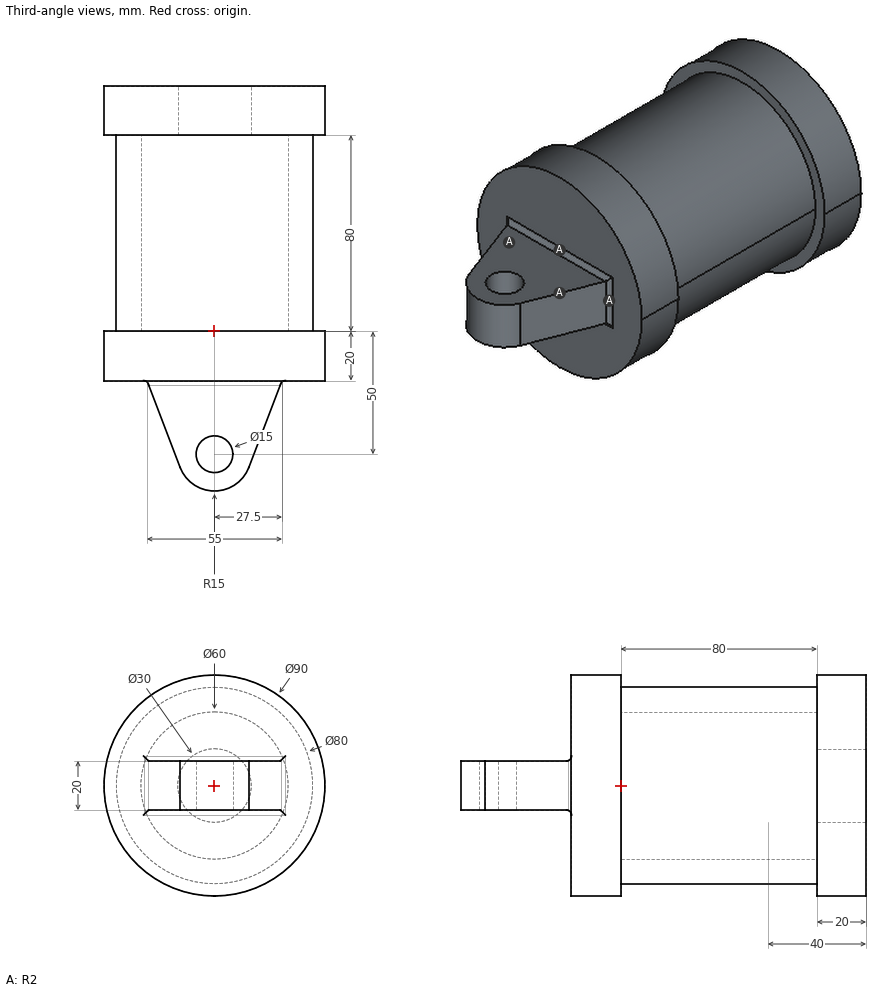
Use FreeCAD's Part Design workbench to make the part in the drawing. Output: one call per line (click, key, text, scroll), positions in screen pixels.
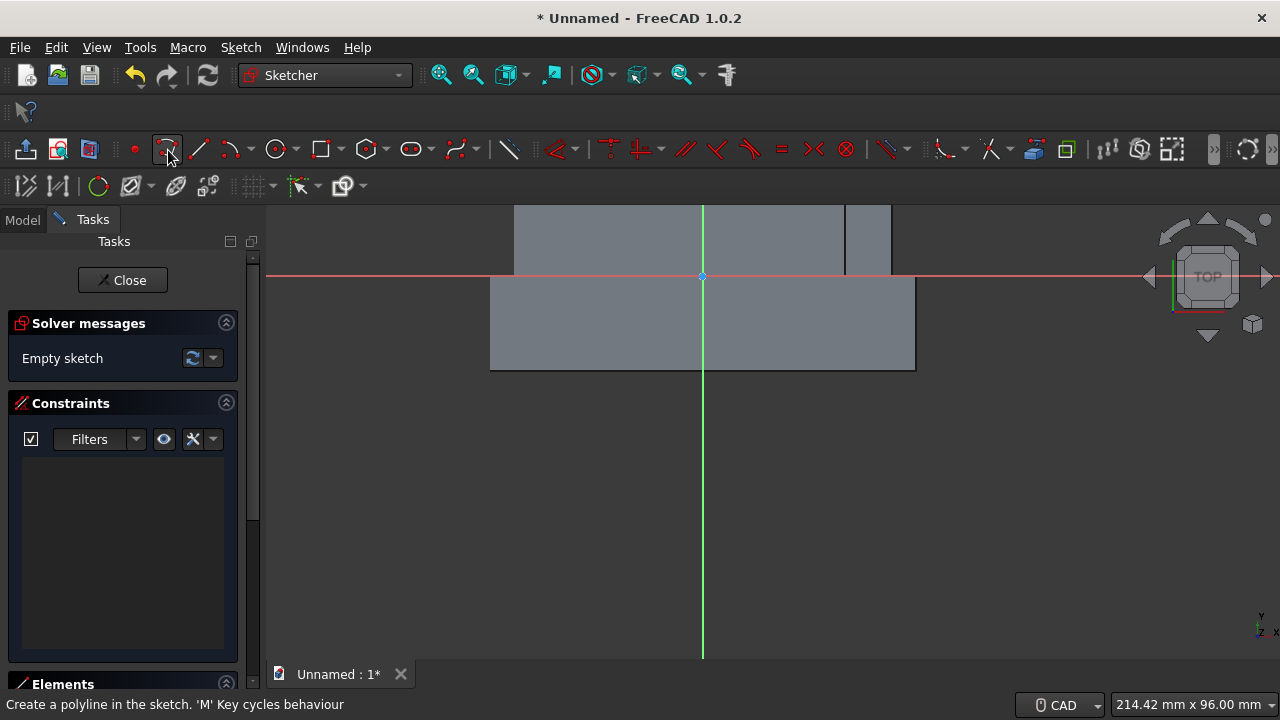
click(769, 538)
click(833, 371)
click(573, 371)
click(636, 538)
right_click(636, 538)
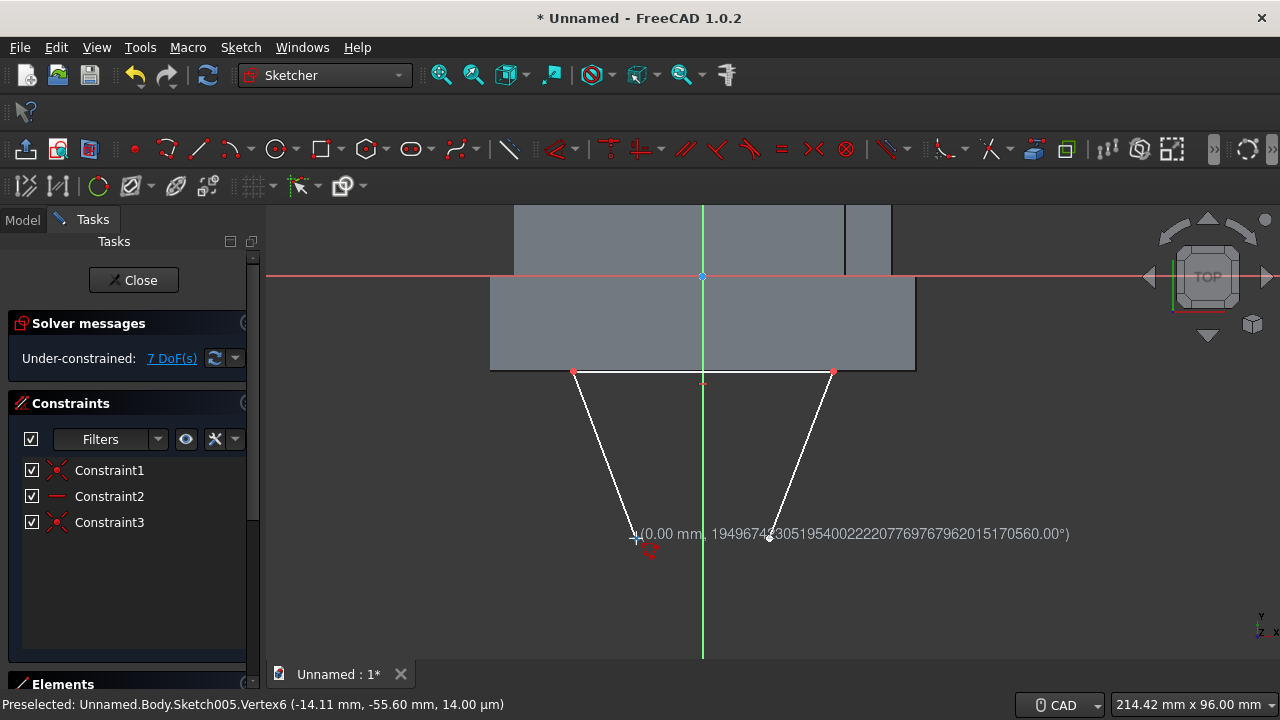
key(g)
key(3)
key(a)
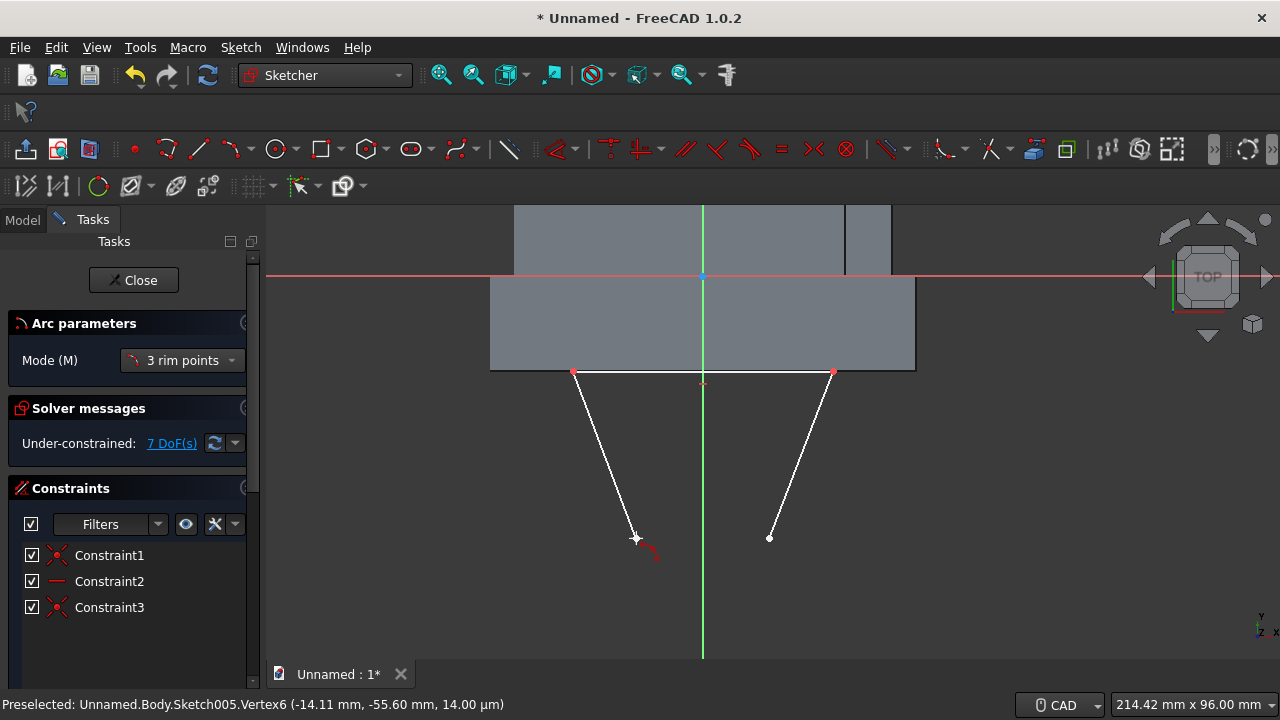
click(636, 539)
click(769, 539)
click(686, 581)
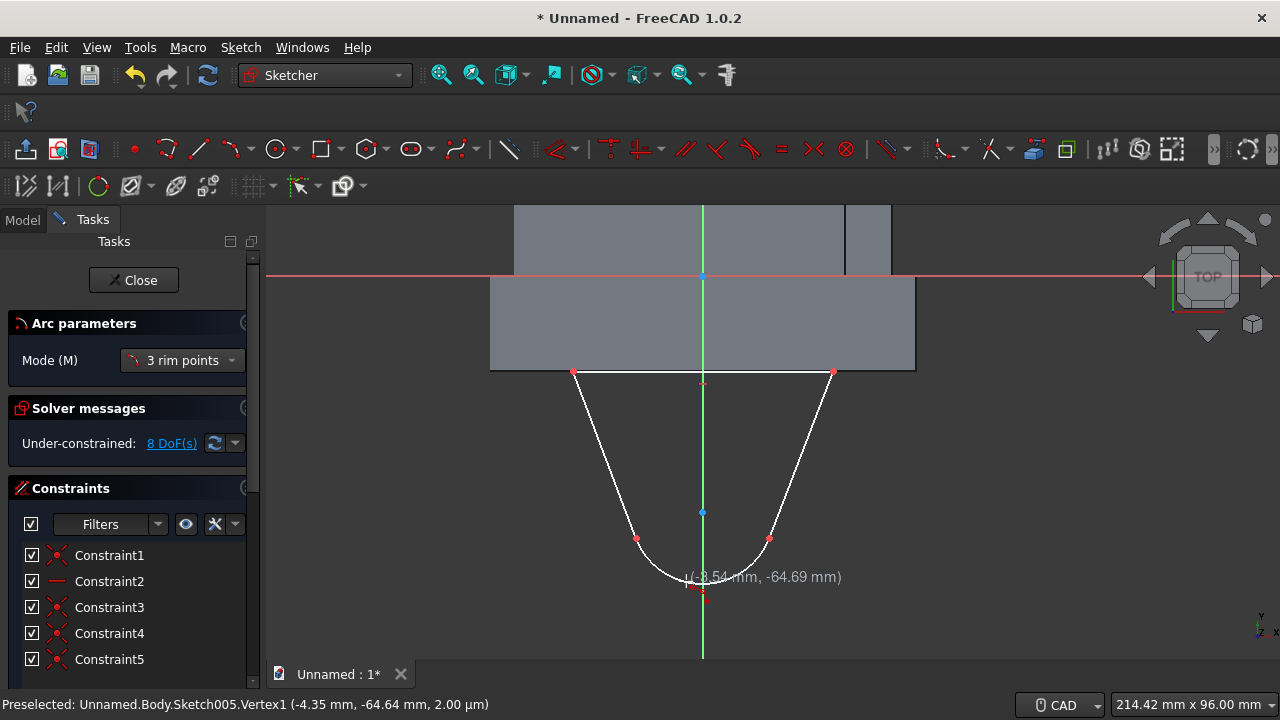
key(g)
key(c)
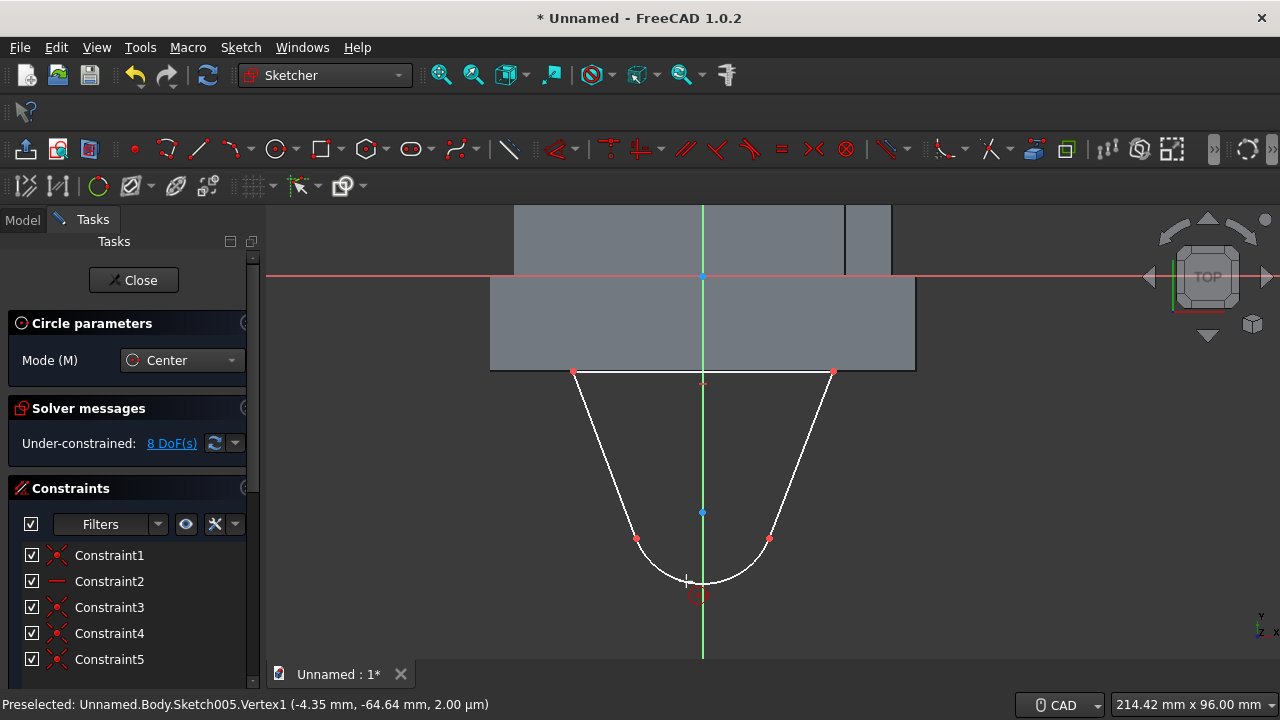
click(703, 513)
move(728, 487)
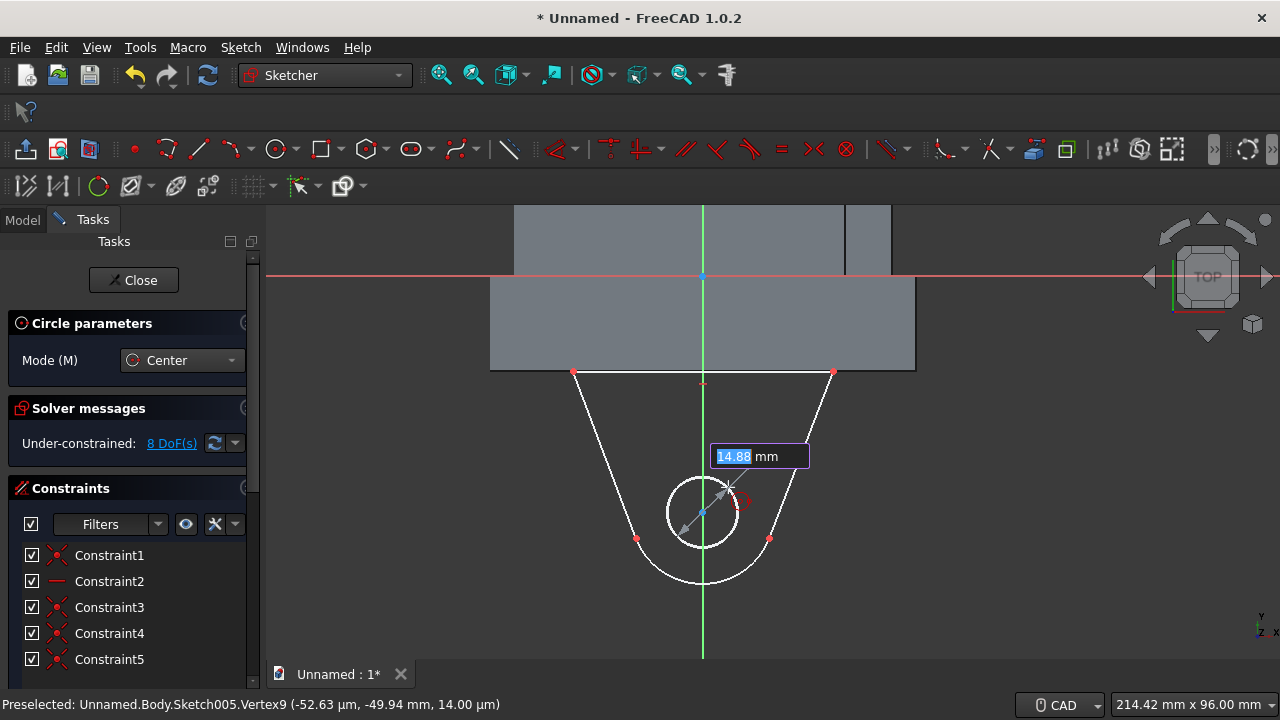
text(15)
key(Return)
key(Escape)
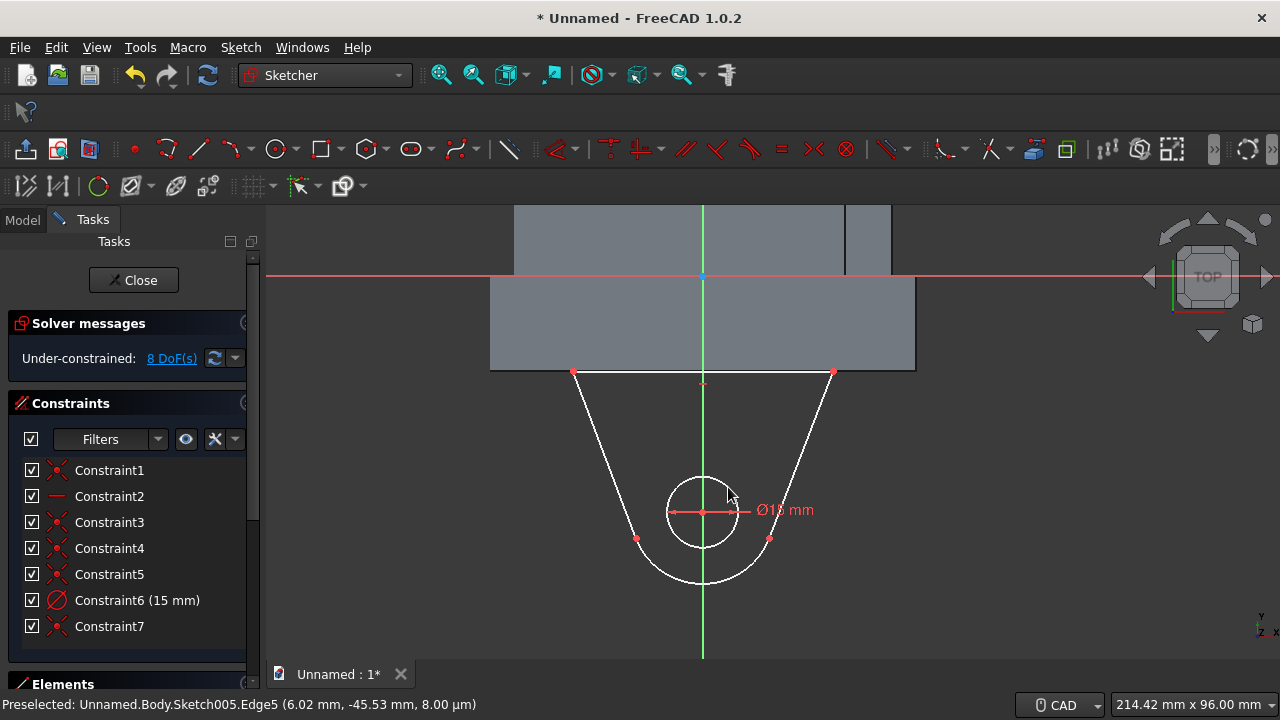
click(788, 489)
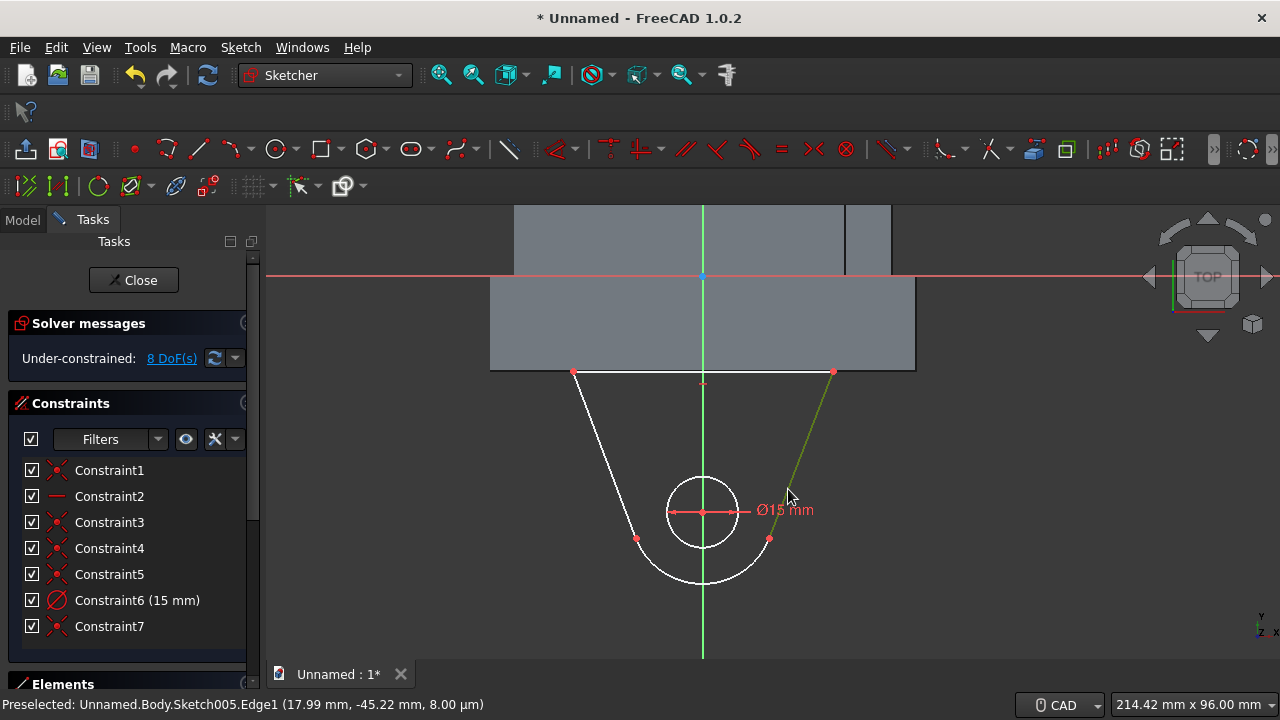
click(670, 576)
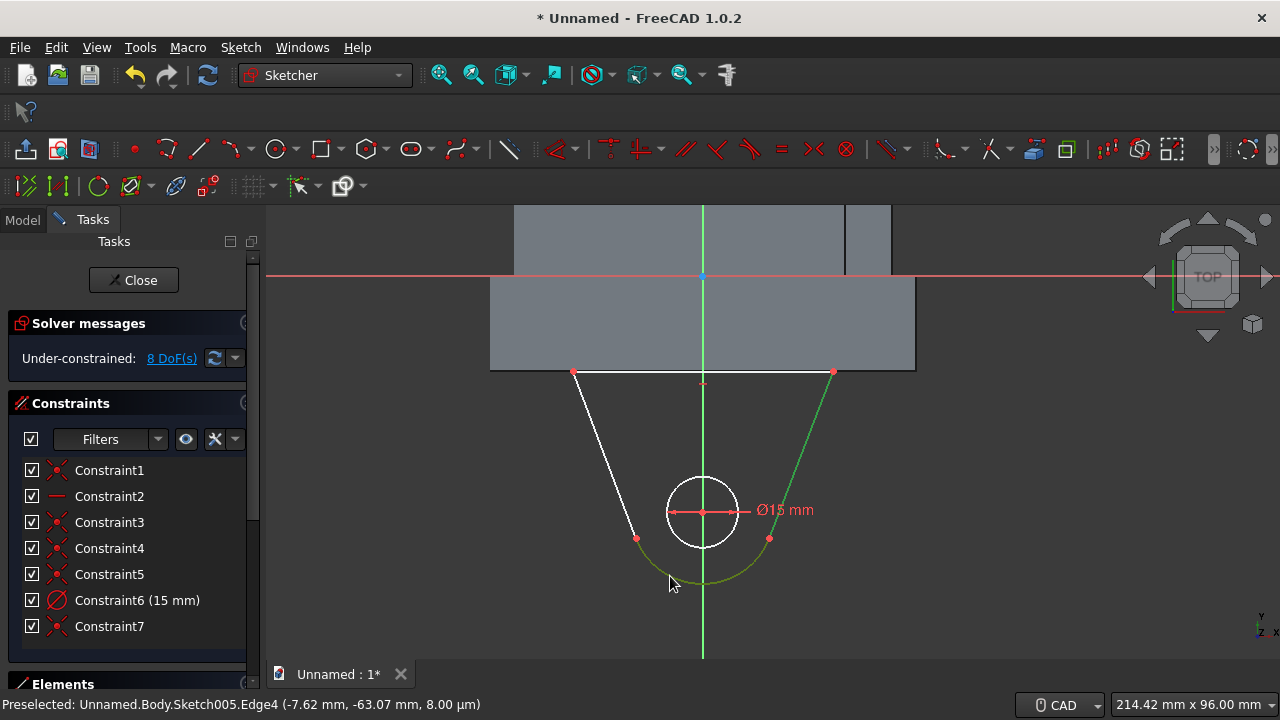
key(t)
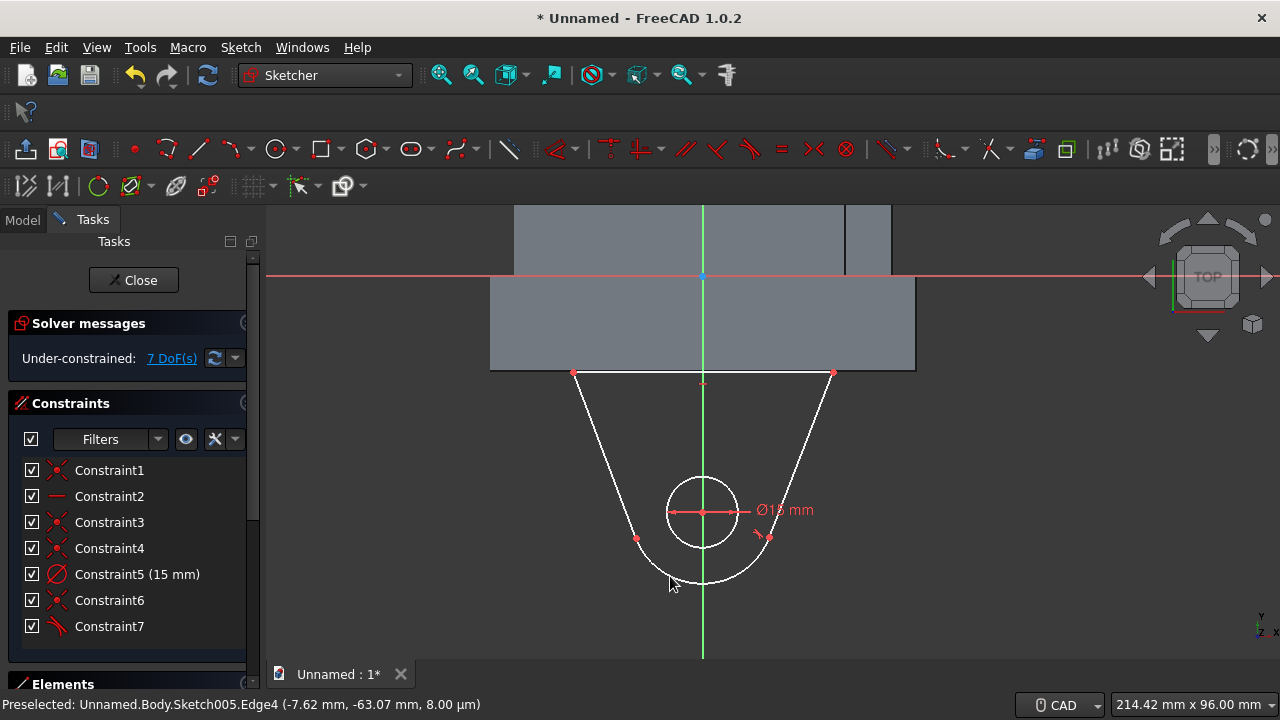
click(592, 422)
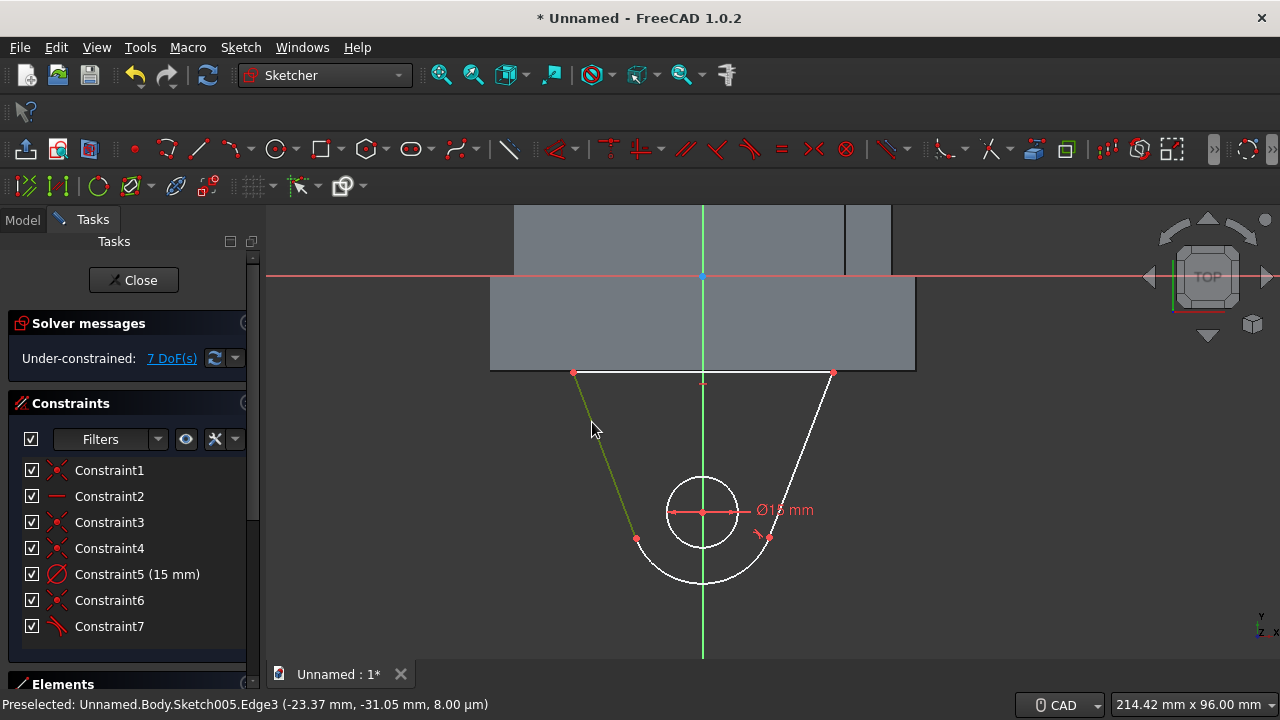
click(670, 576)